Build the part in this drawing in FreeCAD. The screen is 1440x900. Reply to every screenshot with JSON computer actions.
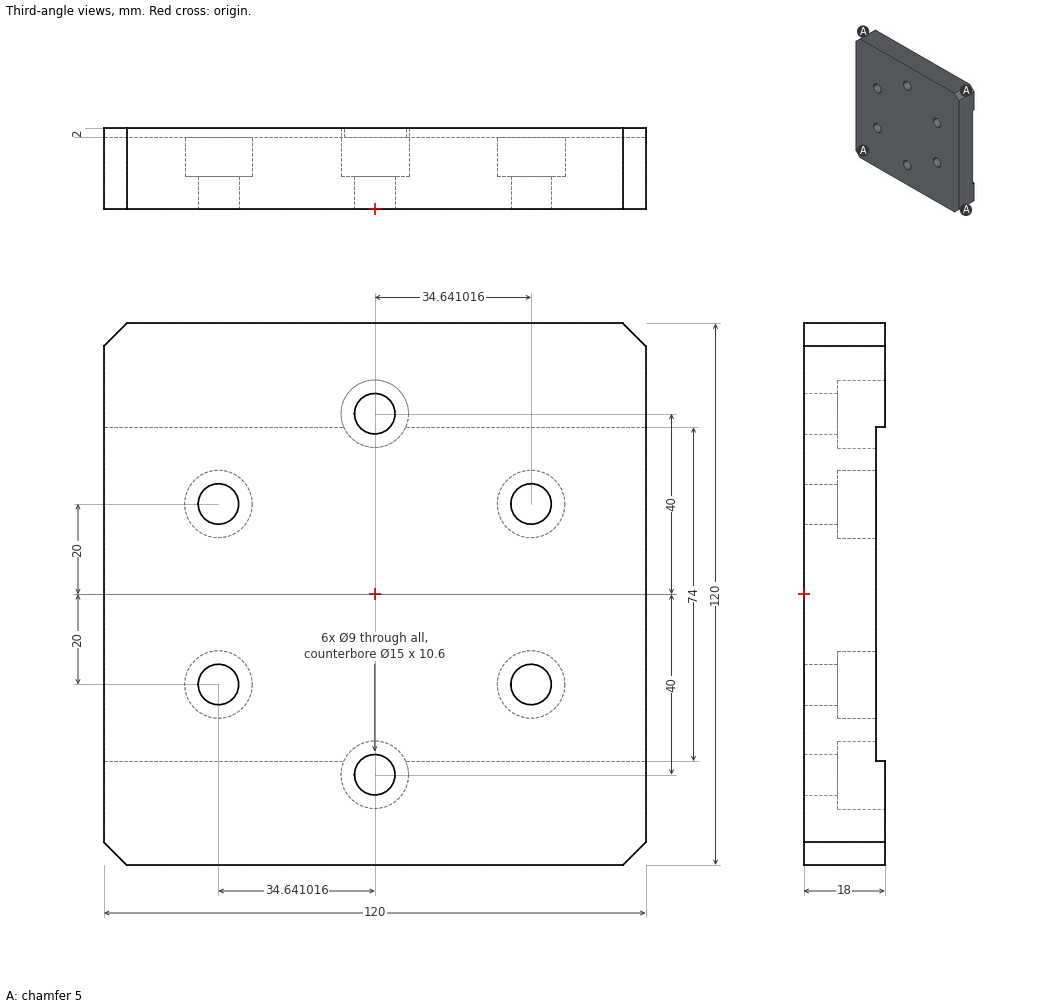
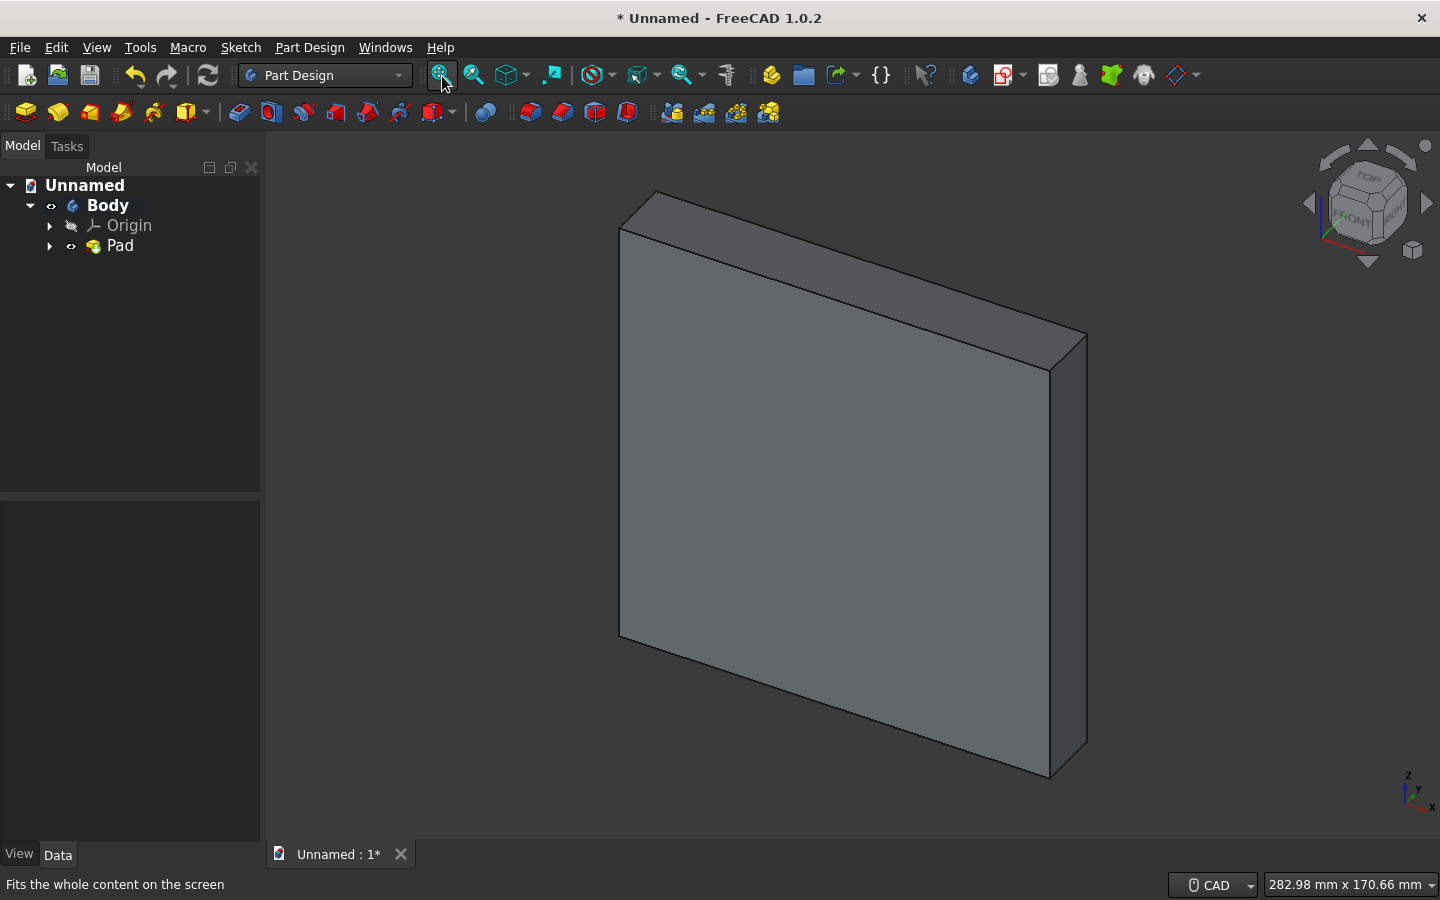
{"action": "key", "text": "4"}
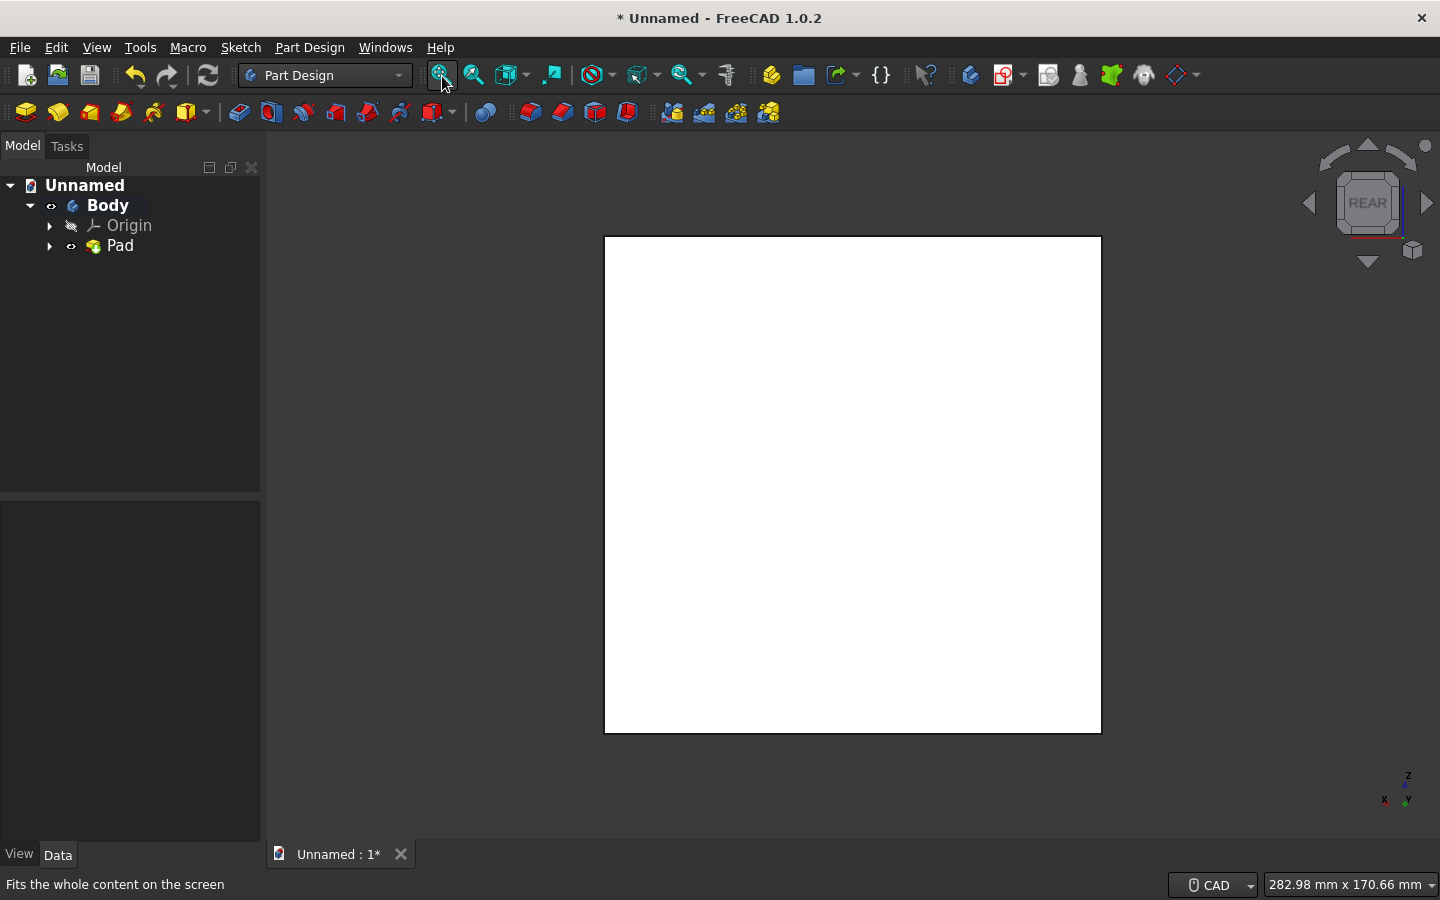
{"action": "left_click", "coordinate": [853, 484]}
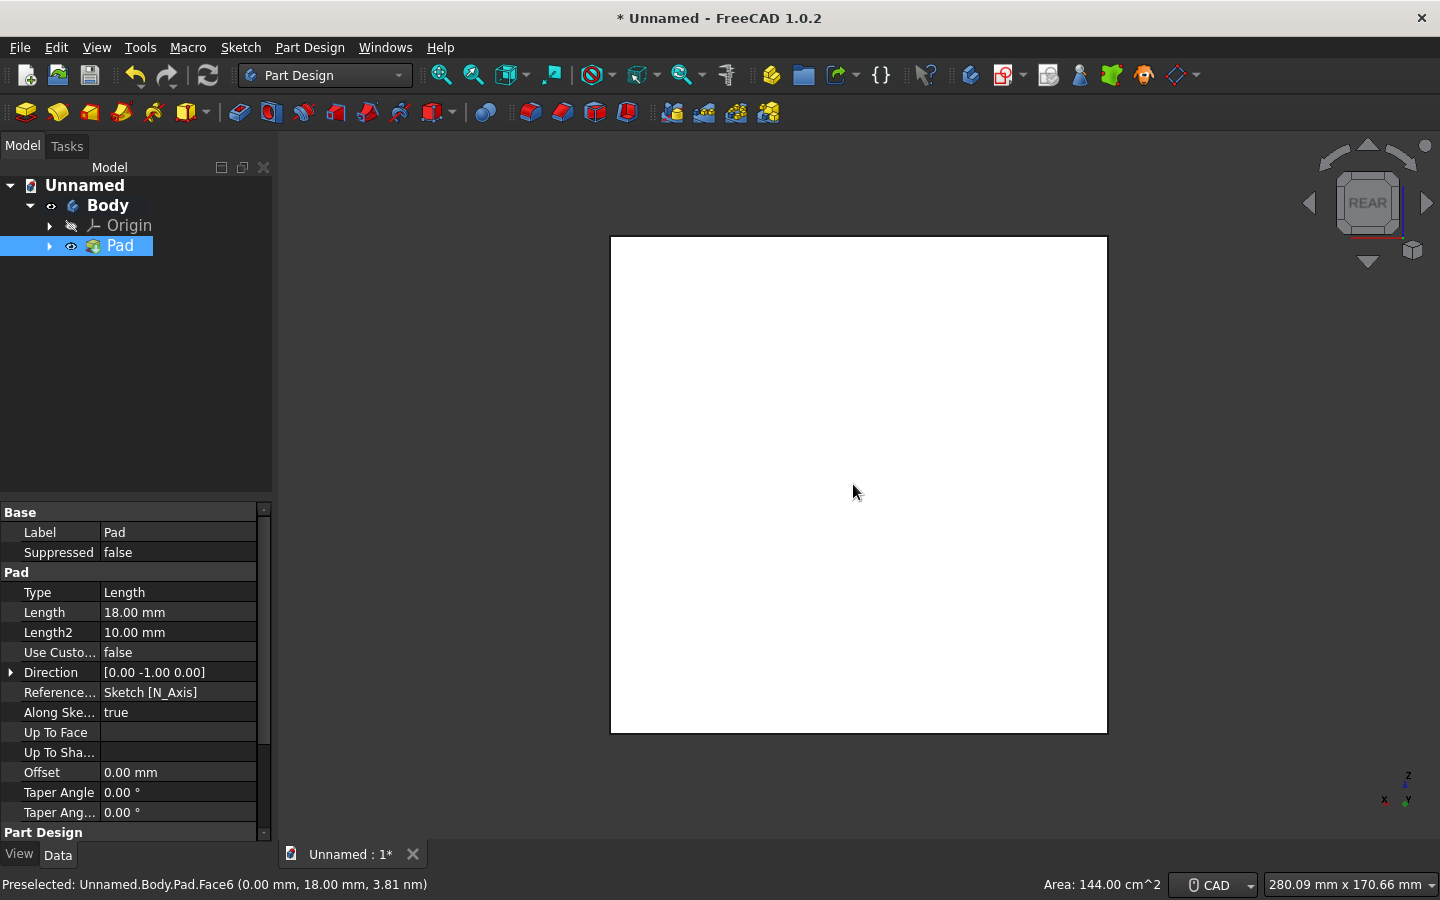
{"action": "left_click", "coordinate": [1004, 76]}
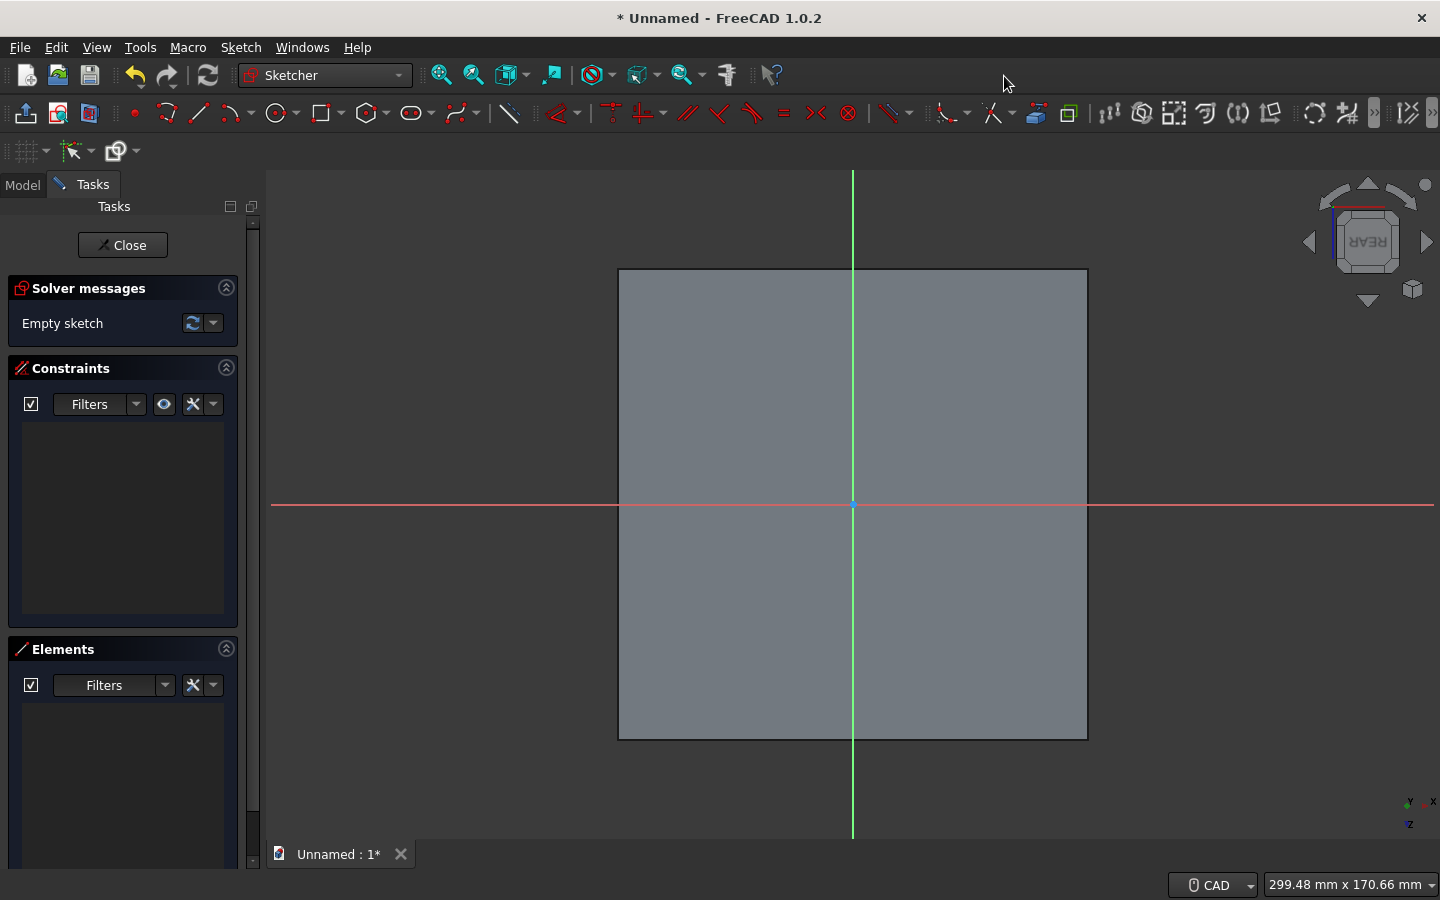
{"action": "left_click", "coordinate": [276, 114]}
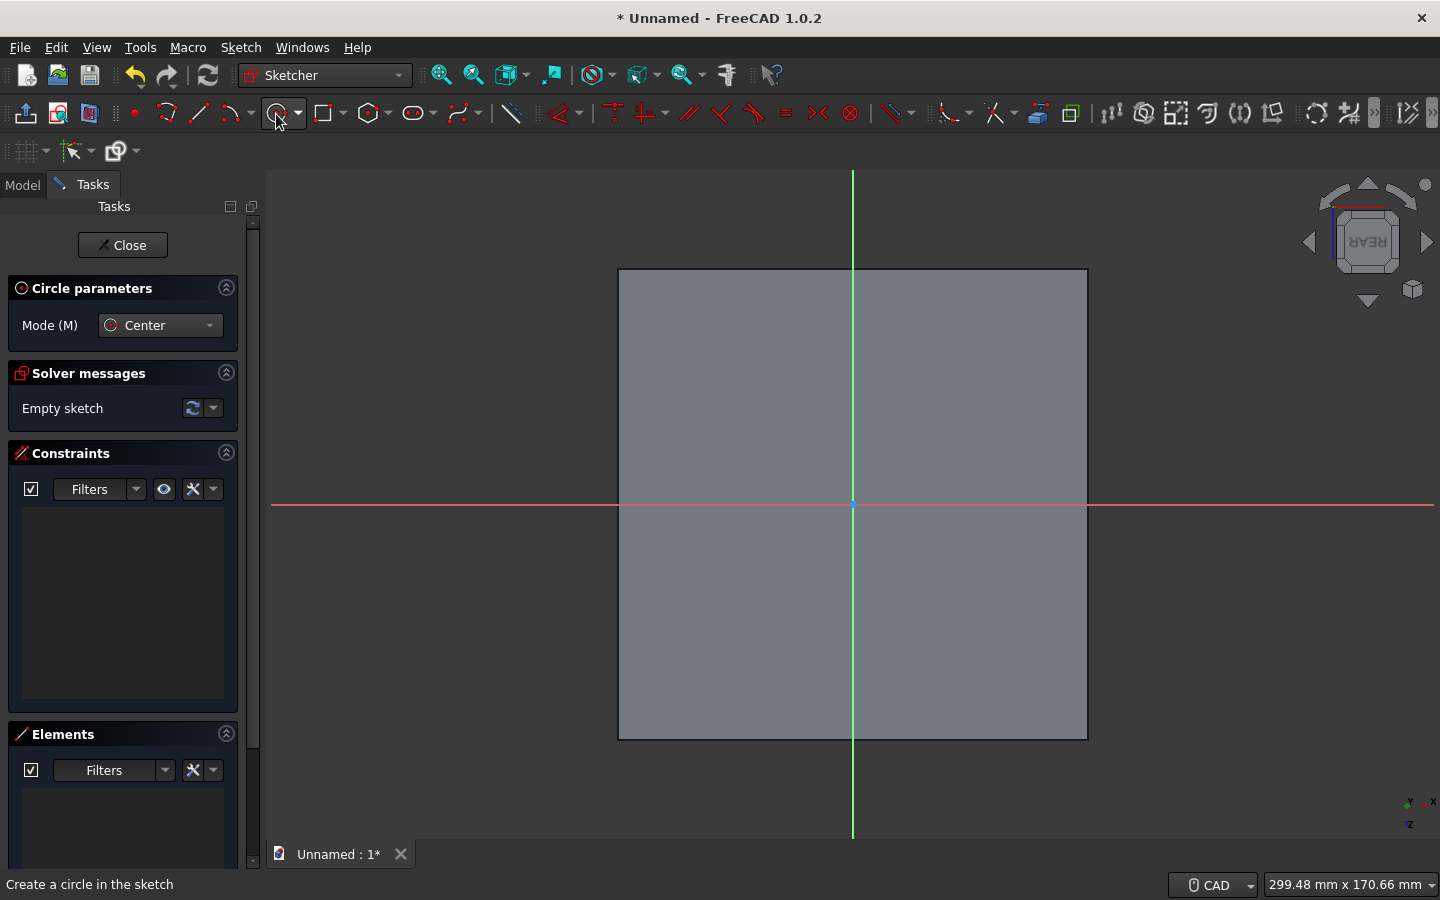
{"action": "scroll", "coordinate": [853, 348], "scroll_direction": "up", "scroll_amount": 2}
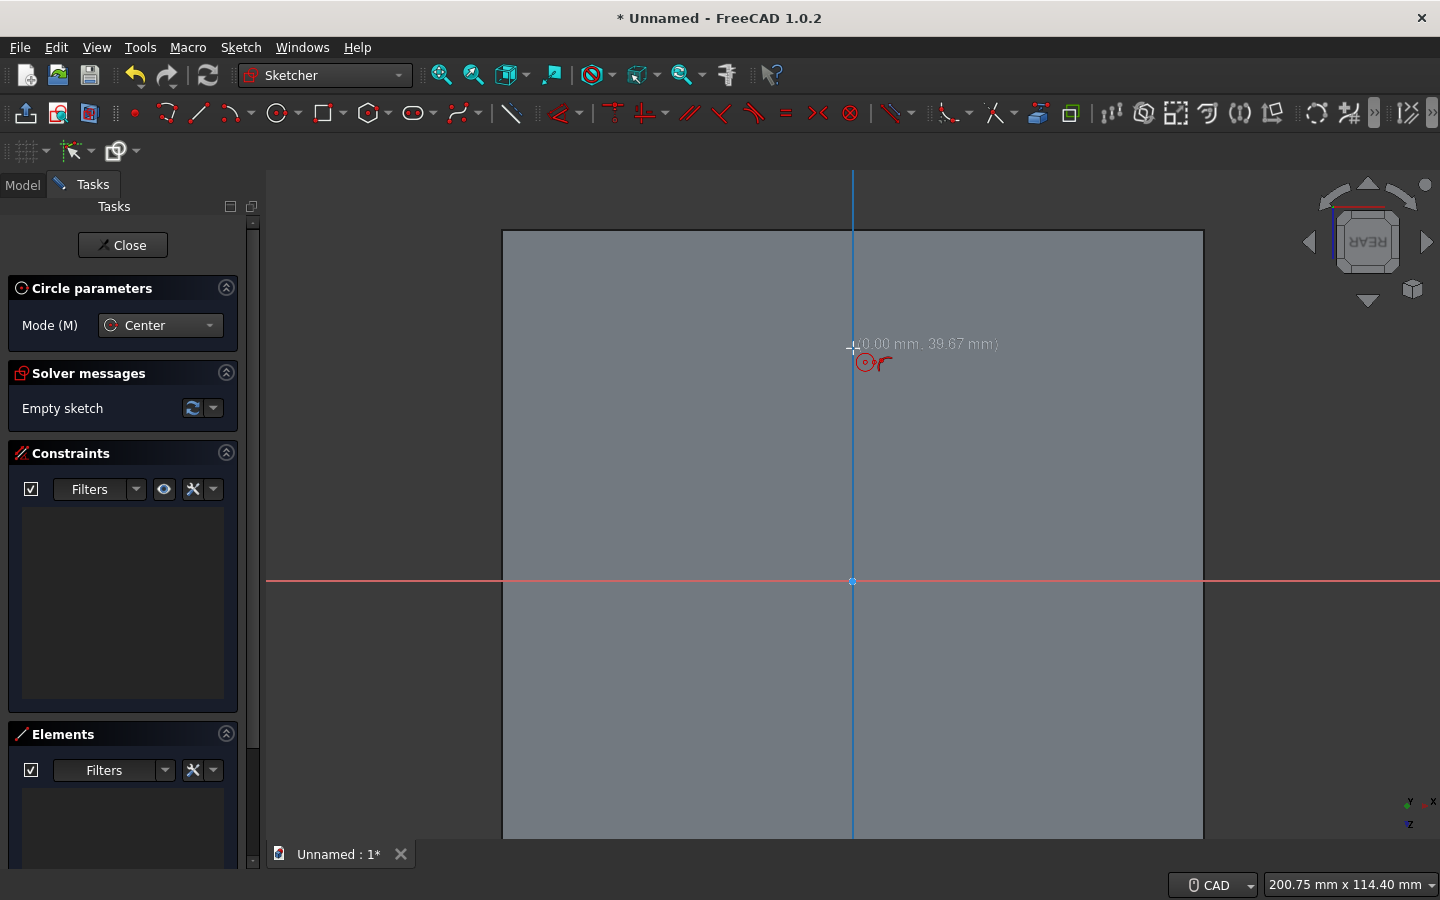
{"action": "left_click", "coordinate": [853, 347]}
{"action": "mouse_move", "coordinate": [871, 329]}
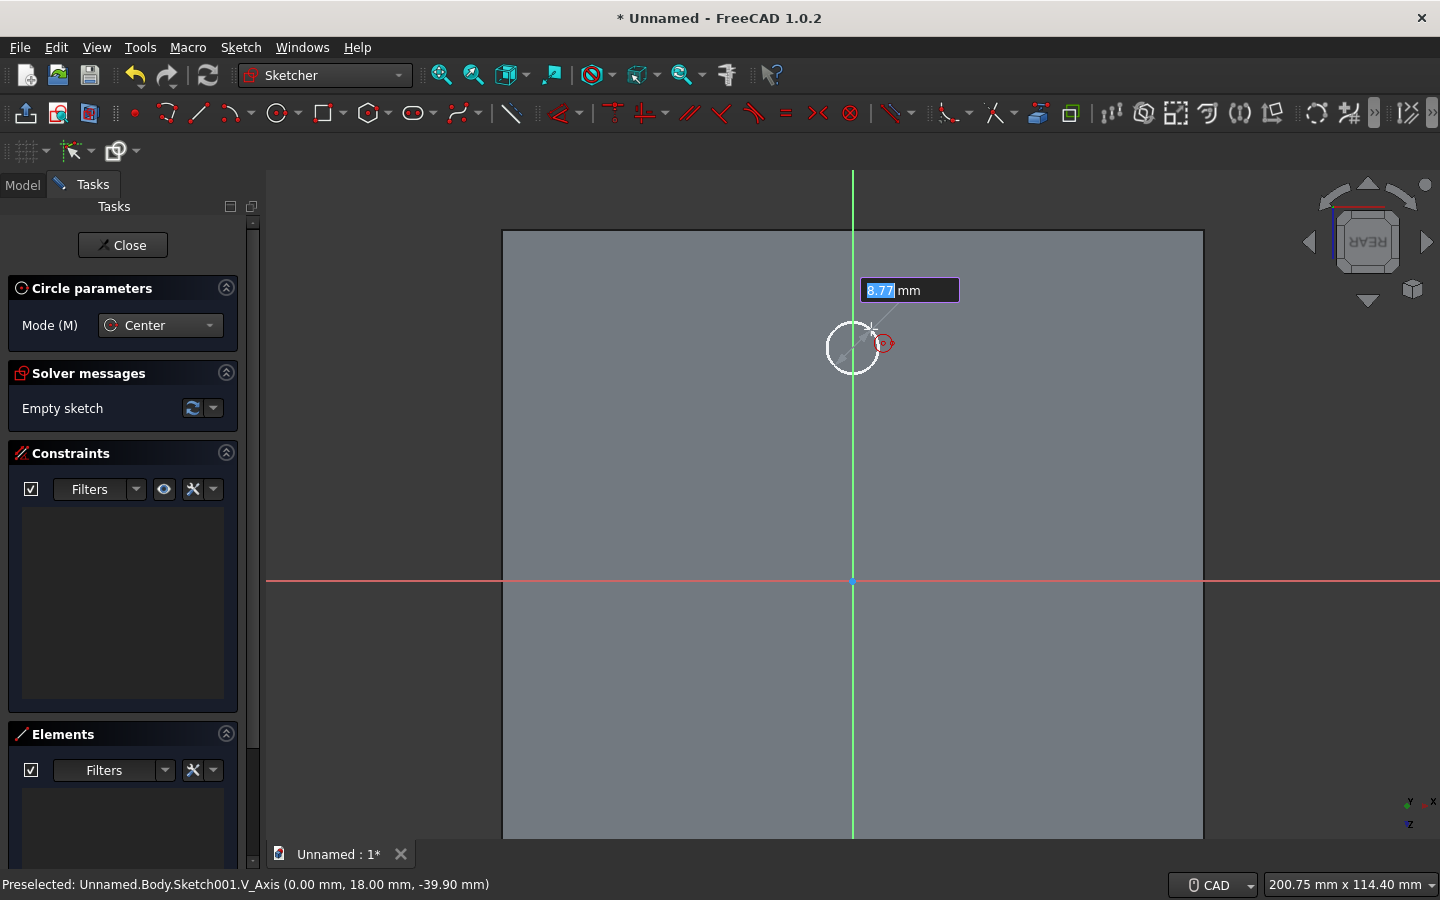
{"action": "type", "text": "9"}
{"action": "key", "text": "Return"}